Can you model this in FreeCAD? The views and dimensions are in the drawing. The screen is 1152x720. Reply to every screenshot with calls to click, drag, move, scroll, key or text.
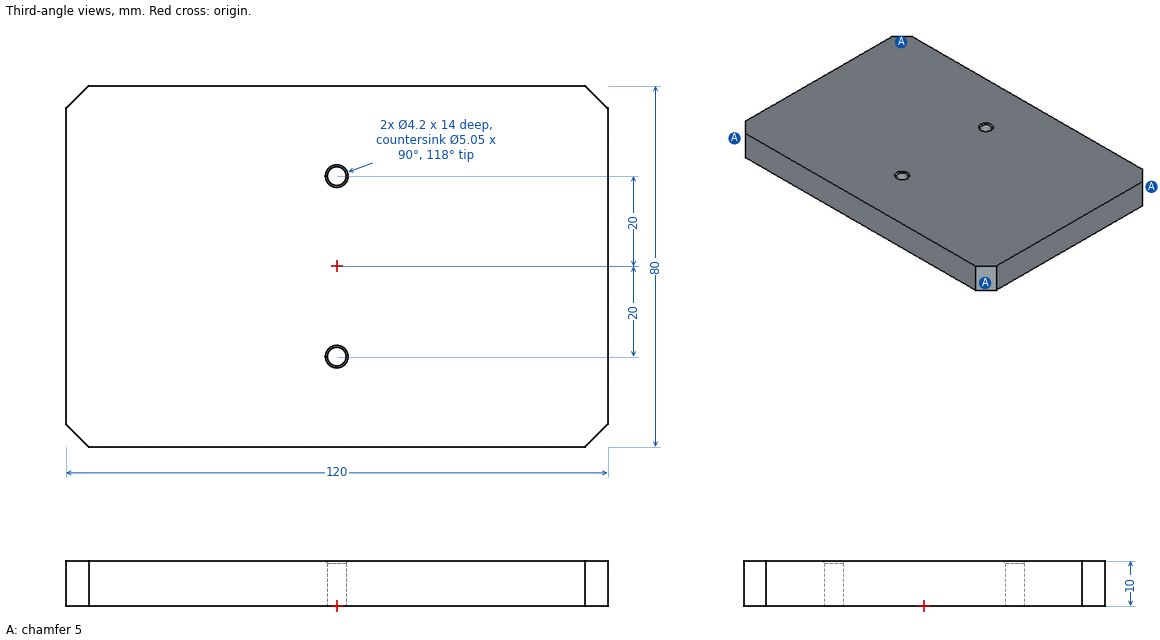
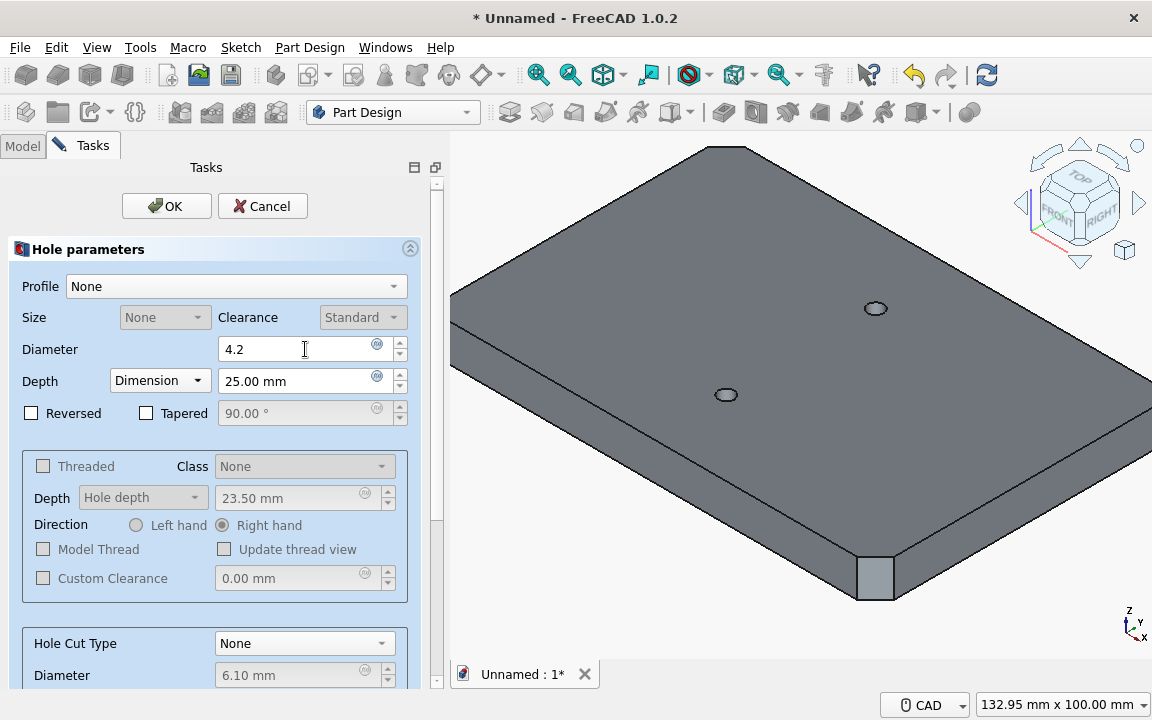
triple_click(305, 381)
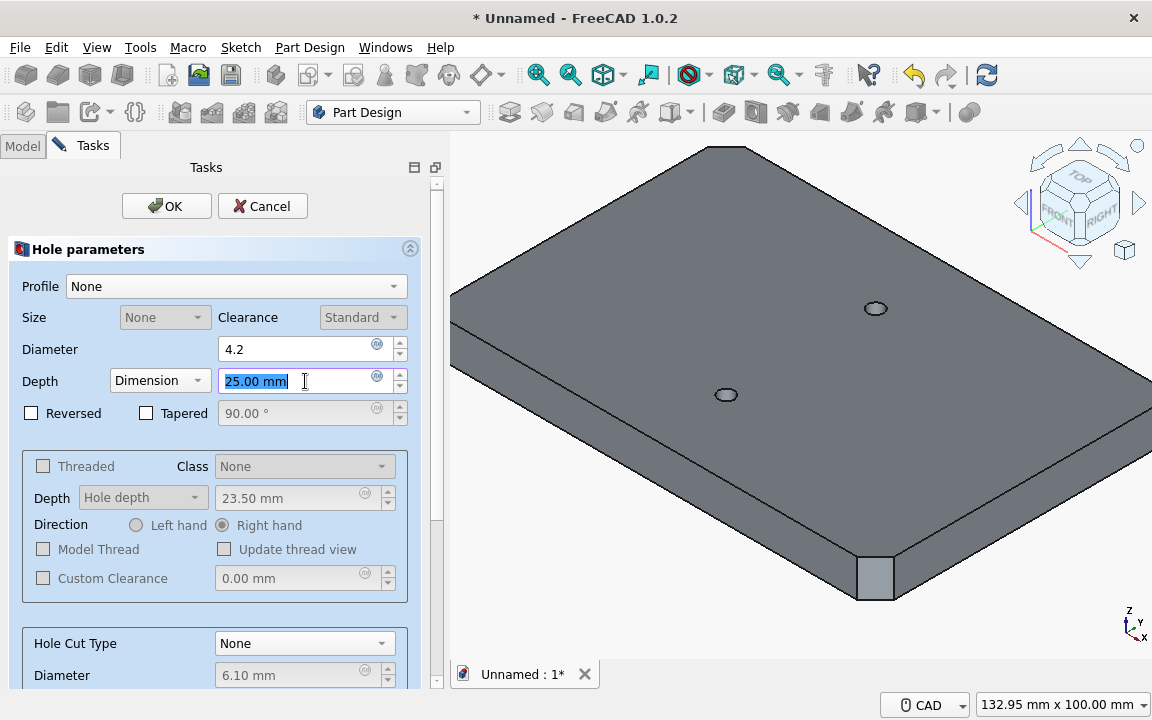
text(14)
key(Tab)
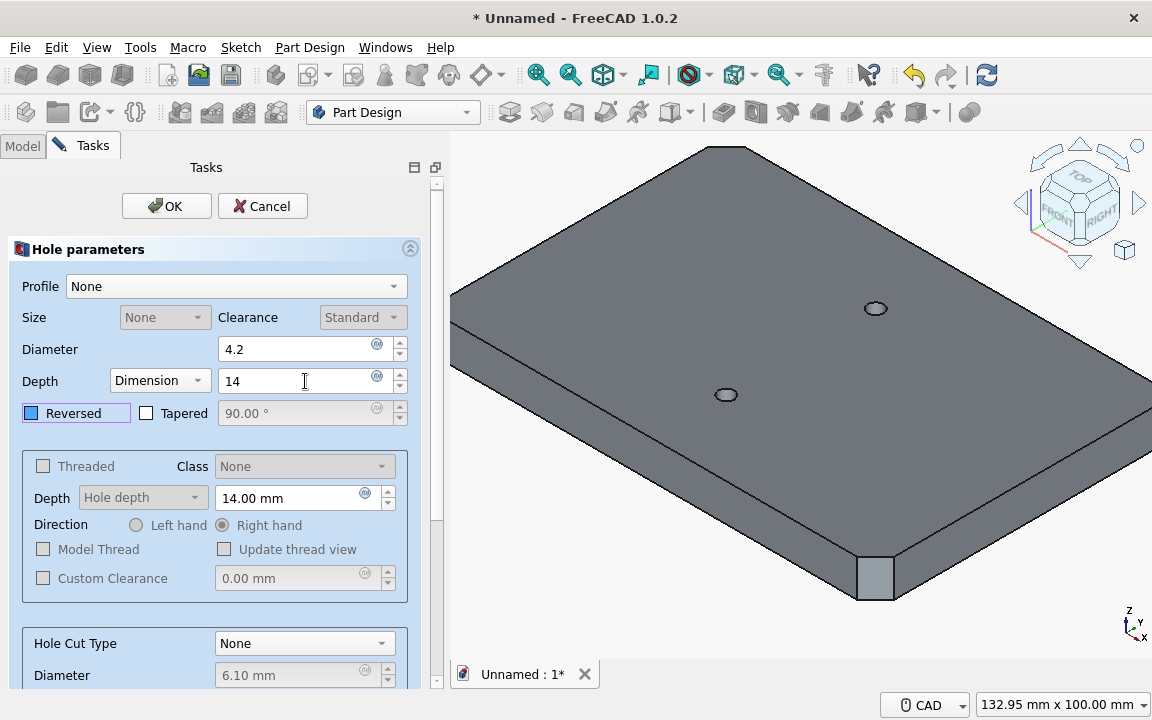
click(306, 644)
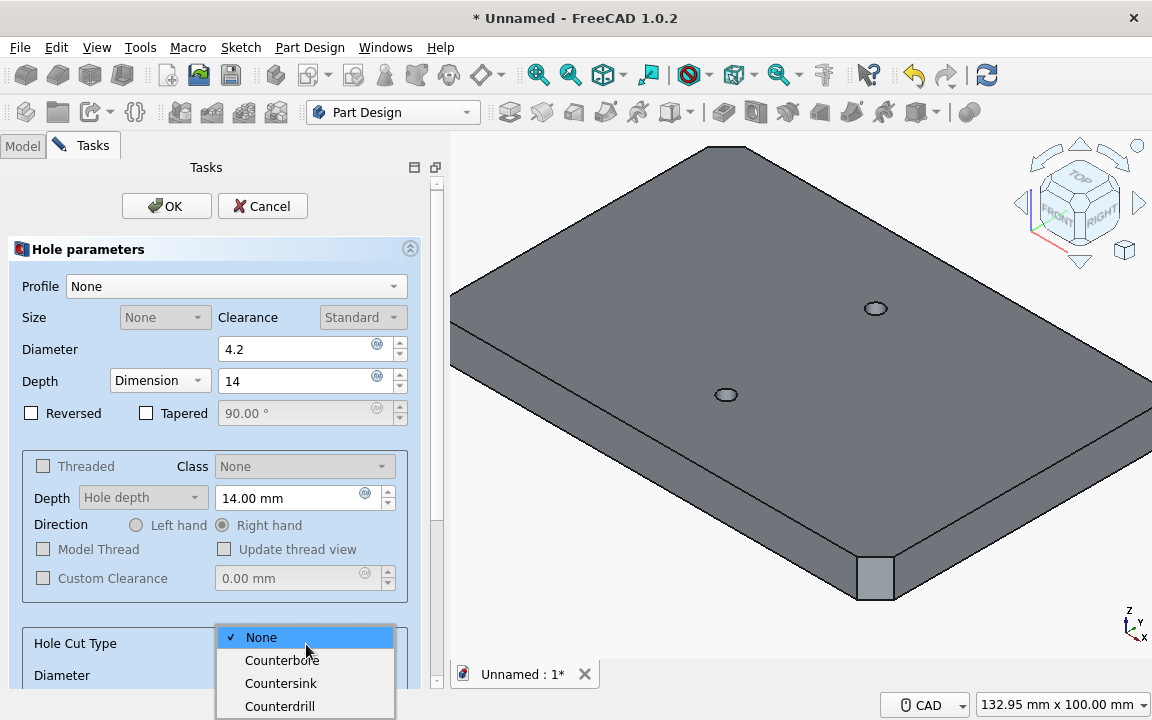
click(304, 684)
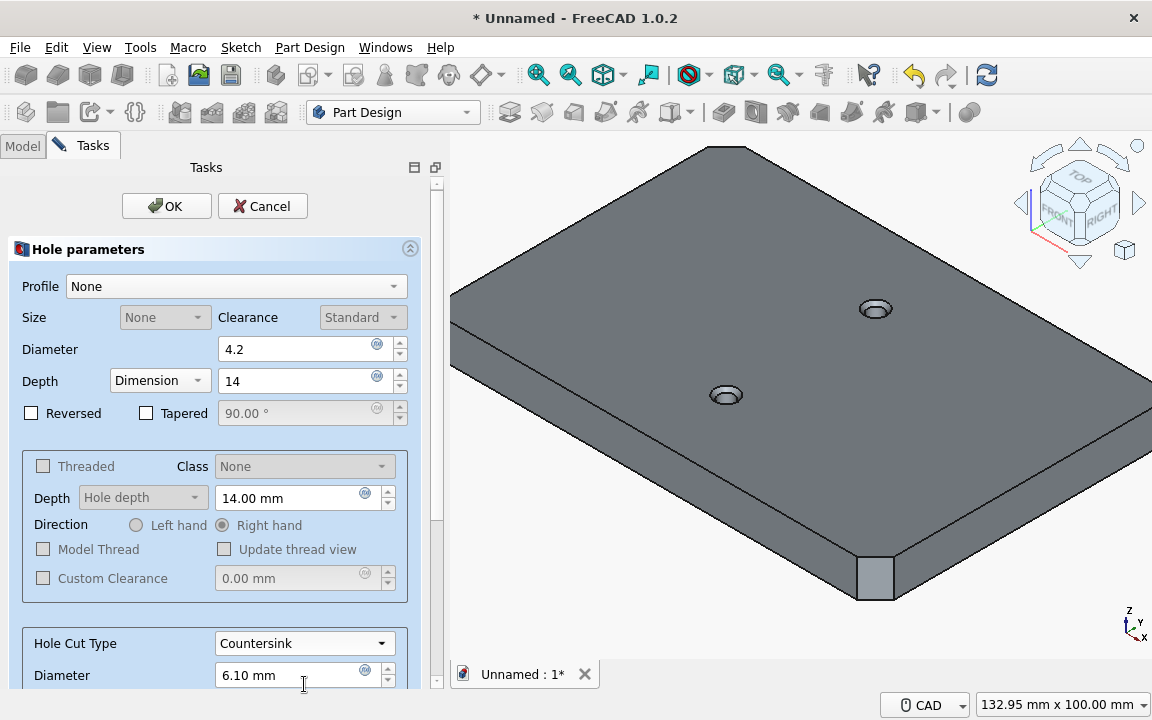
triple_click(298, 675)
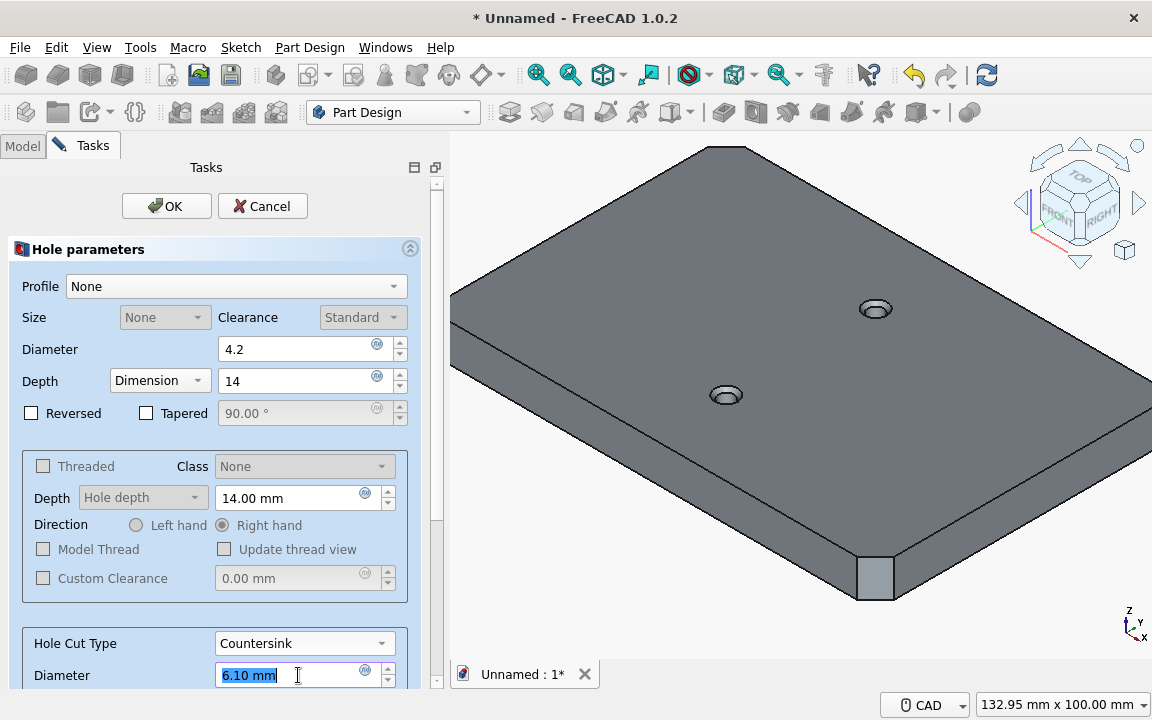
text(5.05)
key(Tab)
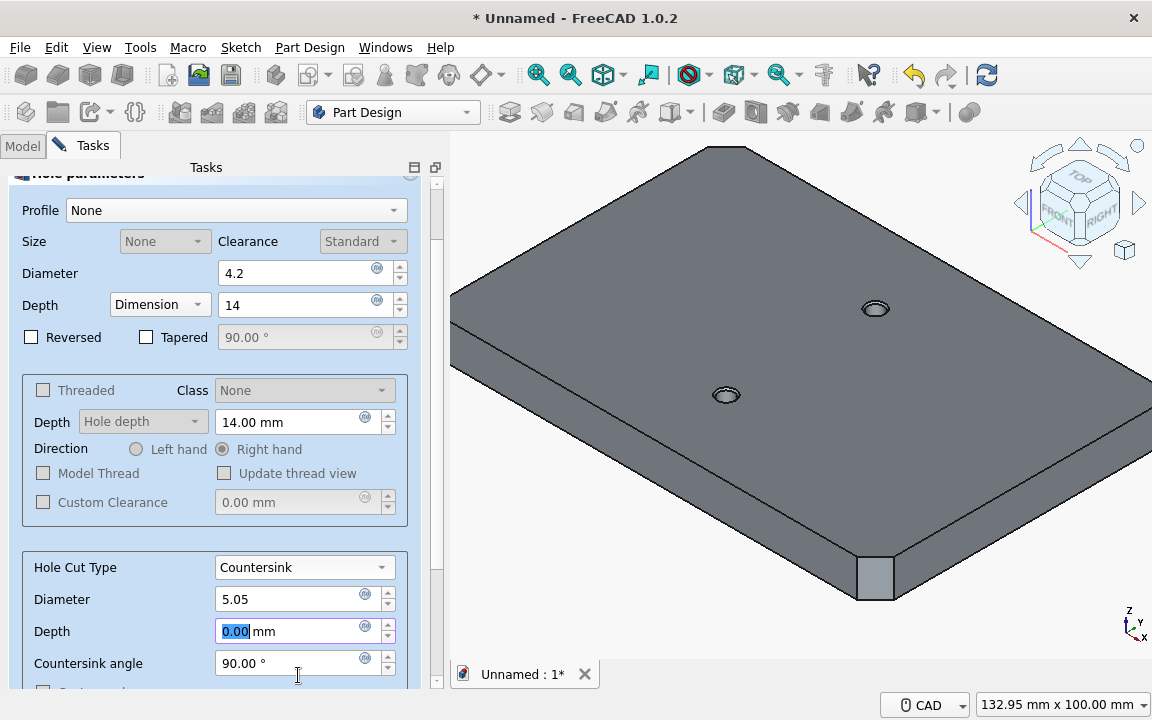
scroll(437, 432, up, 3)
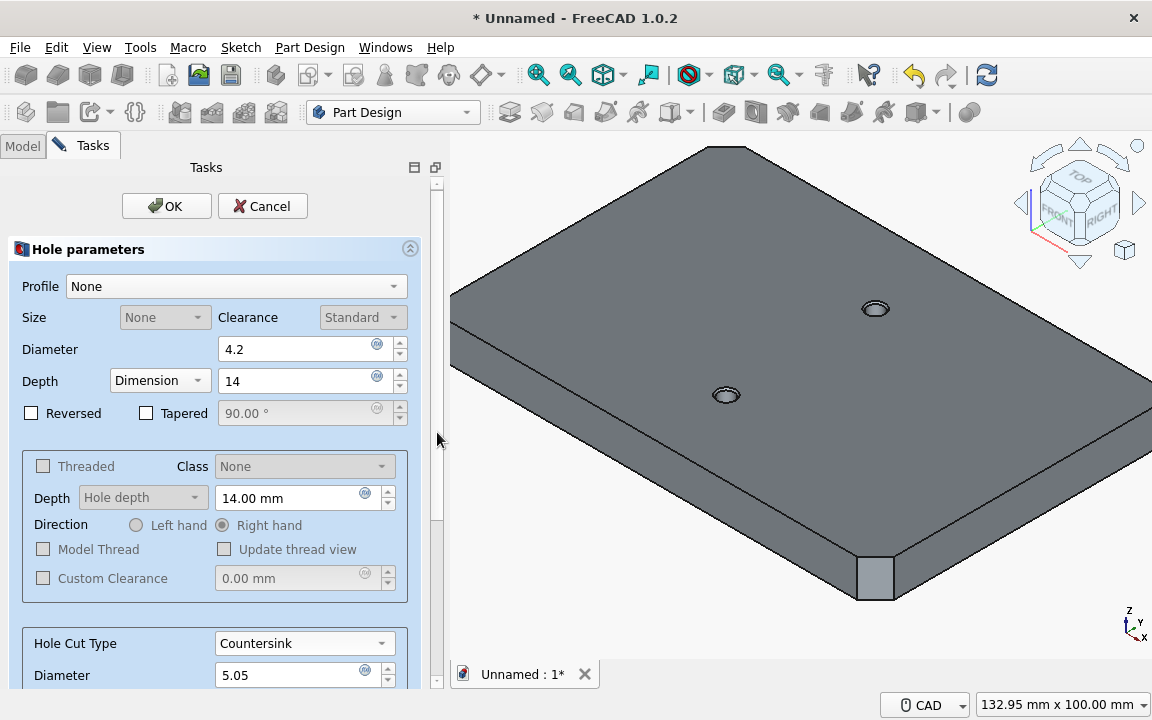
click(167, 206)